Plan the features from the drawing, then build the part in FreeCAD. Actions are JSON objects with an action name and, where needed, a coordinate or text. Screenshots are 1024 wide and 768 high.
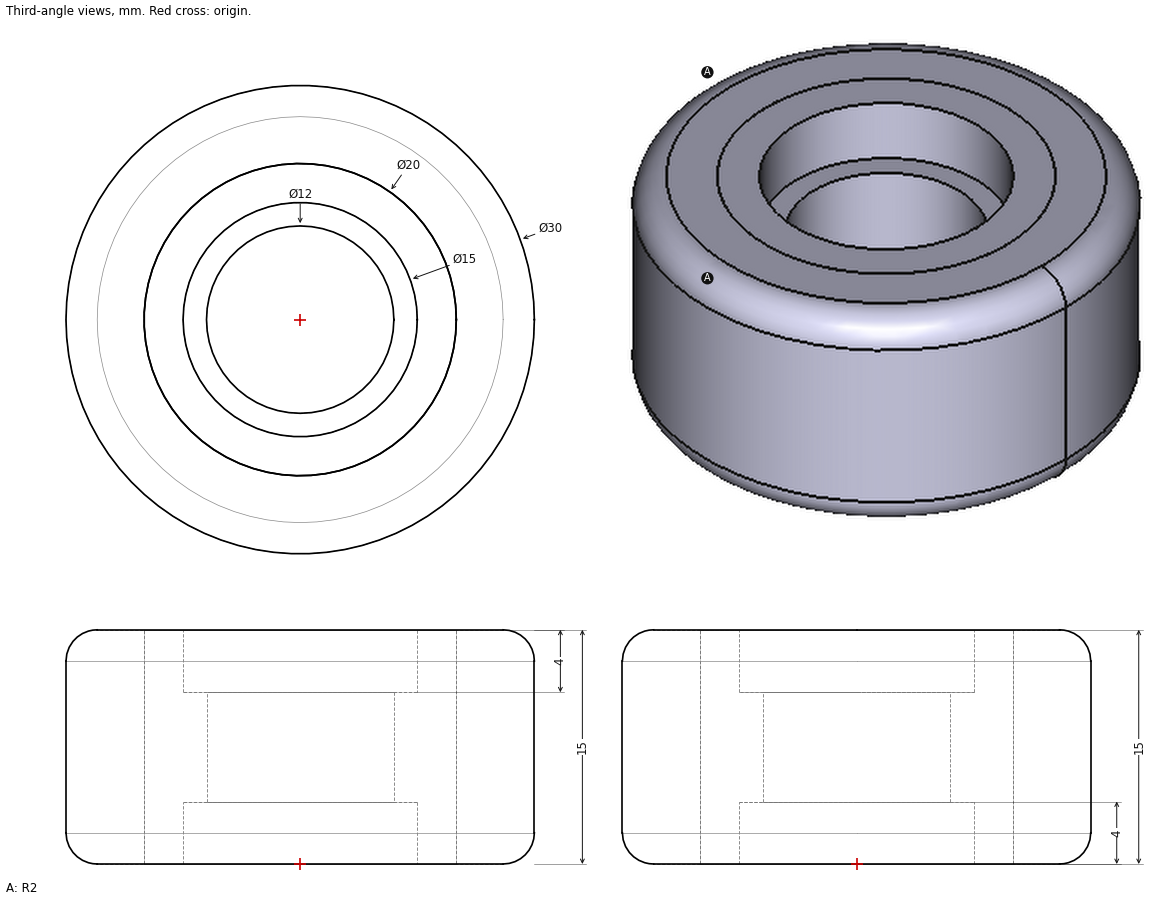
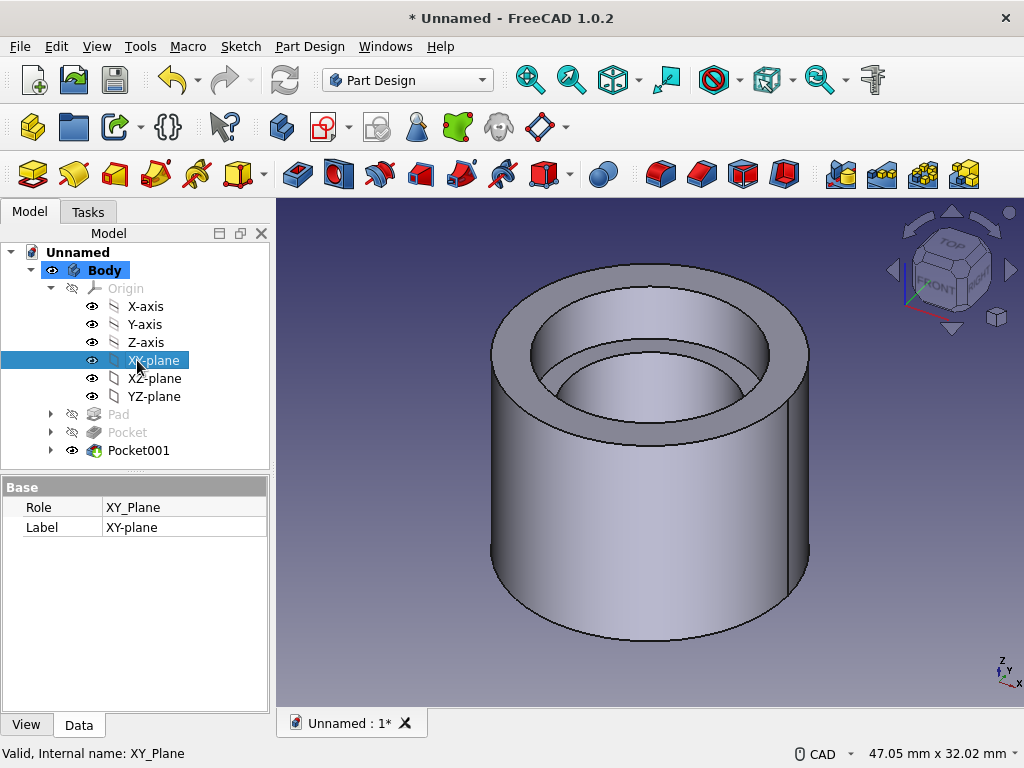
{"action": "left_click", "coordinate": [540, 128]}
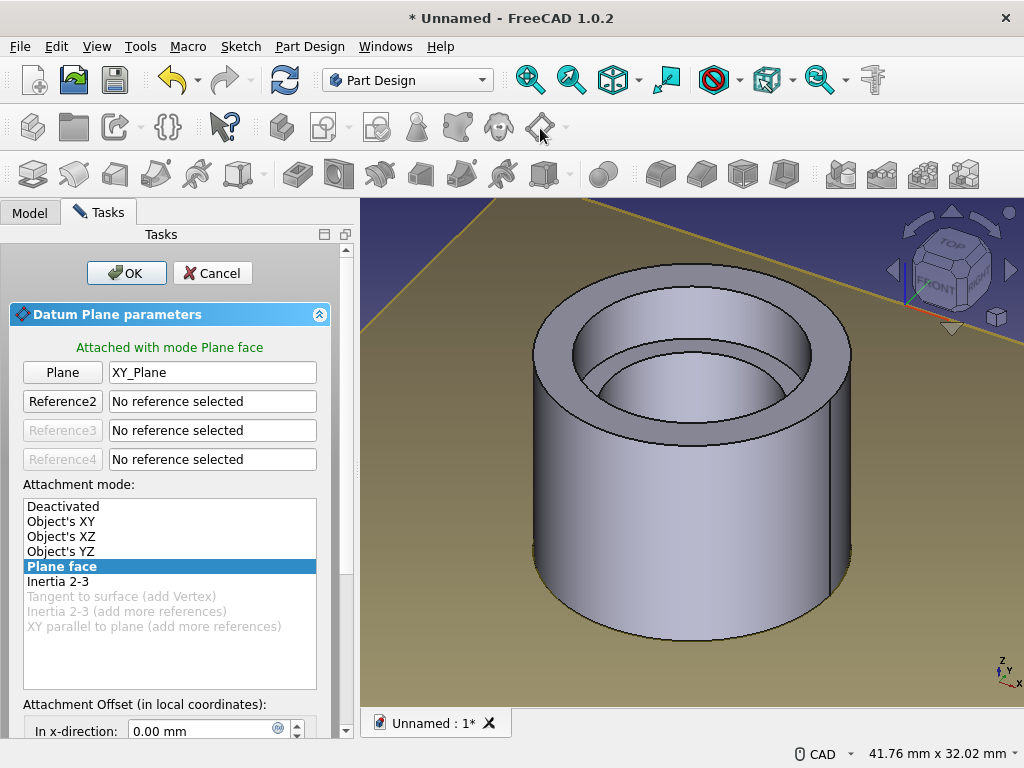
{"action": "scroll", "coordinate": [346, 491], "scroll_direction": "down", "scroll_amount": 3}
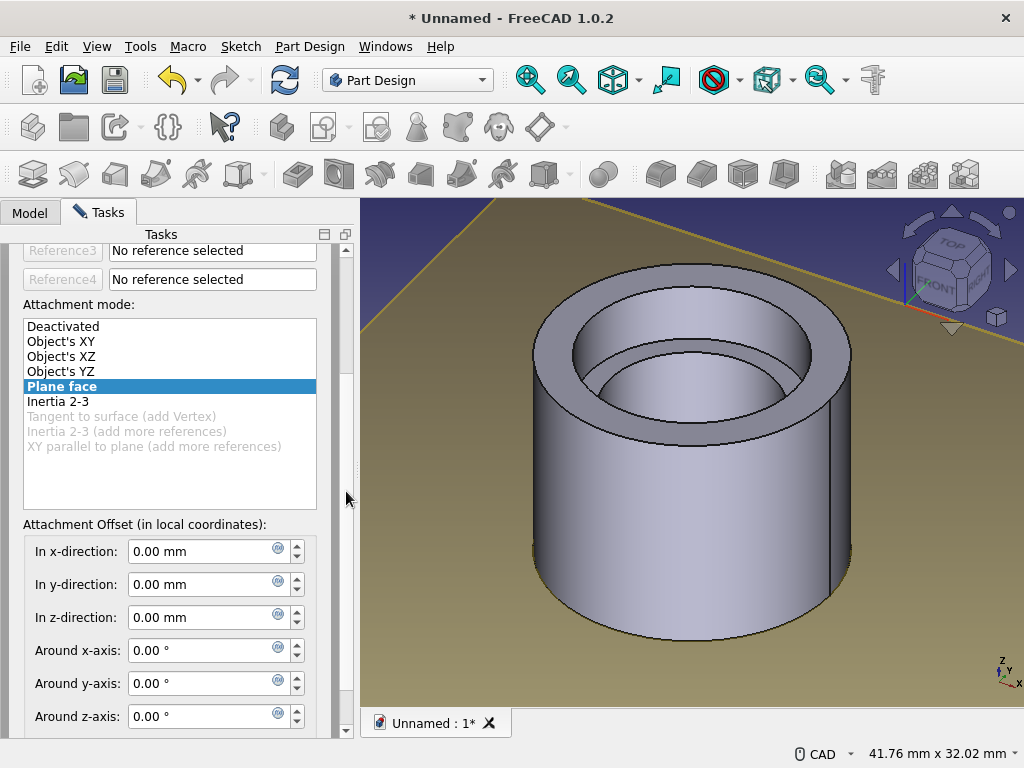
{"action": "triple_click", "coordinate": [210, 618]}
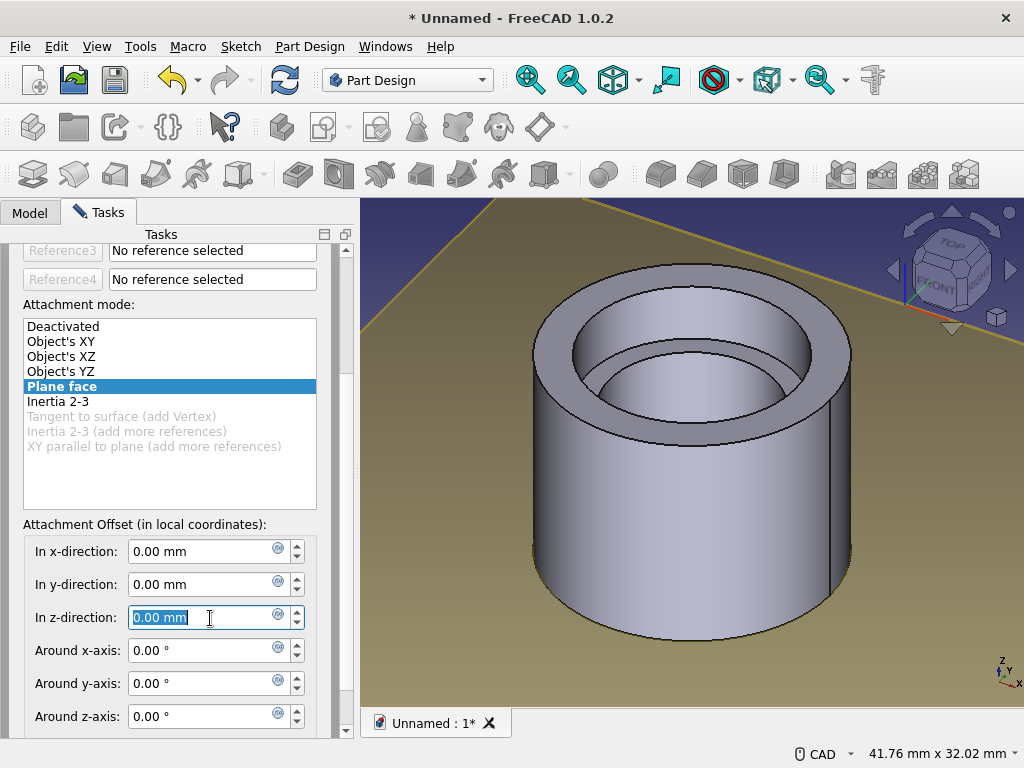
{"action": "type", "text": "4"}
{"action": "key", "text": "Tab"}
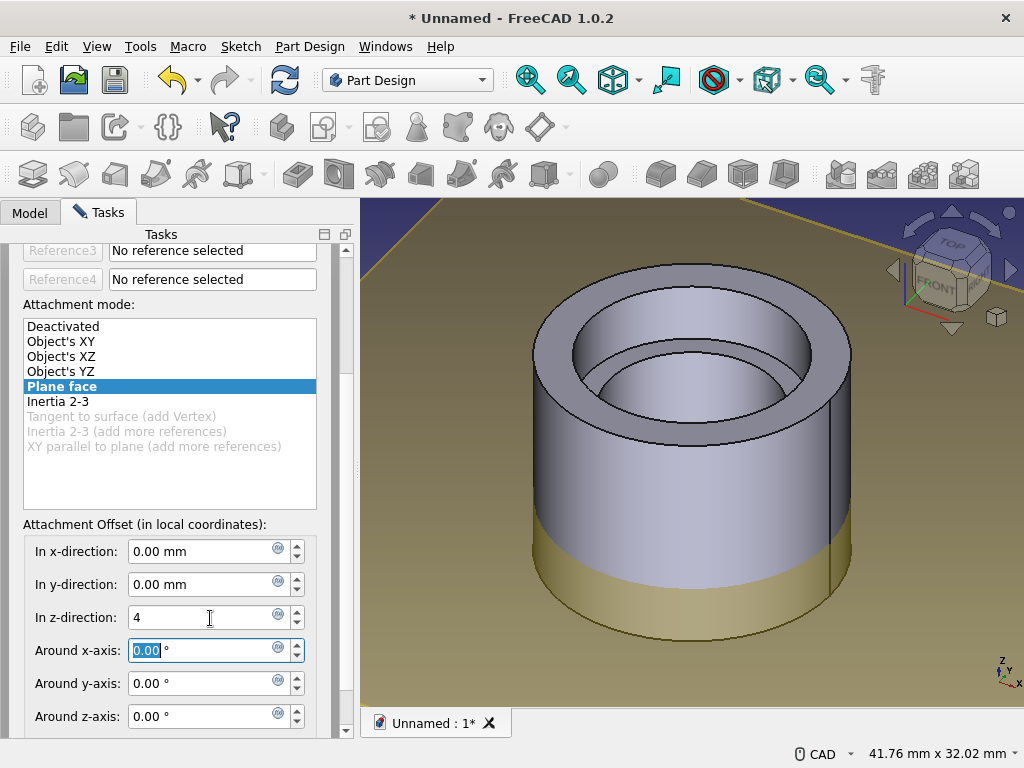
{"action": "scroll", "coordinate": [346, 491], "scroll_direction": "up", "scroll_amount": 4}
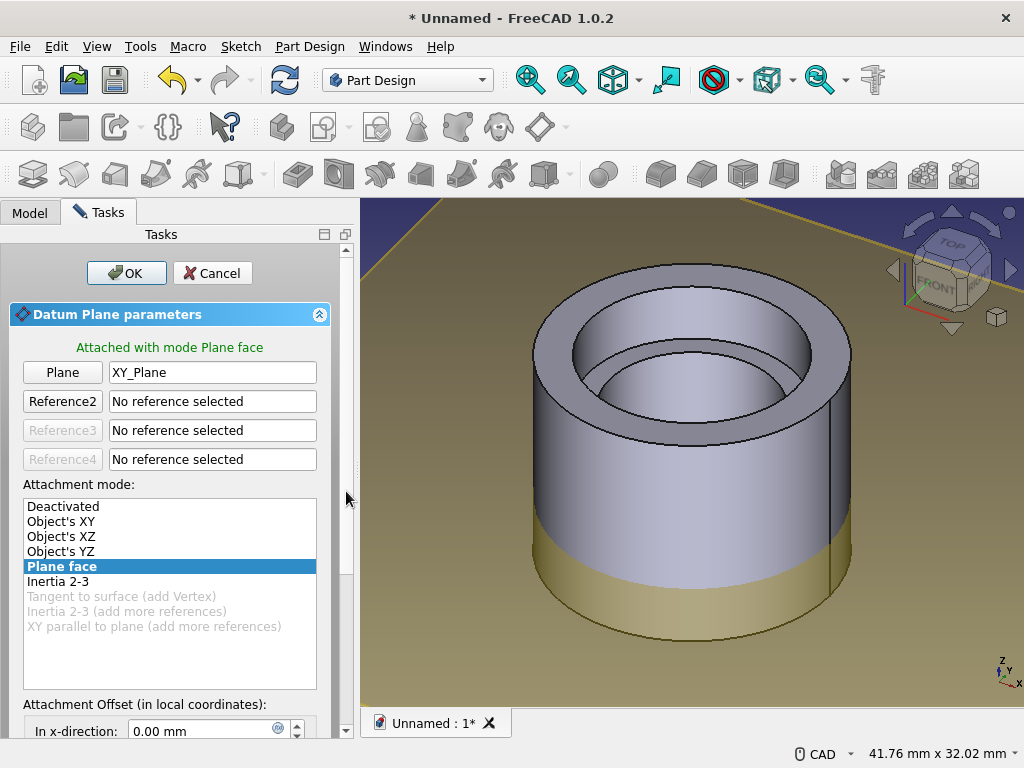
{"action": "left_click", "coordinate": [127, 273]}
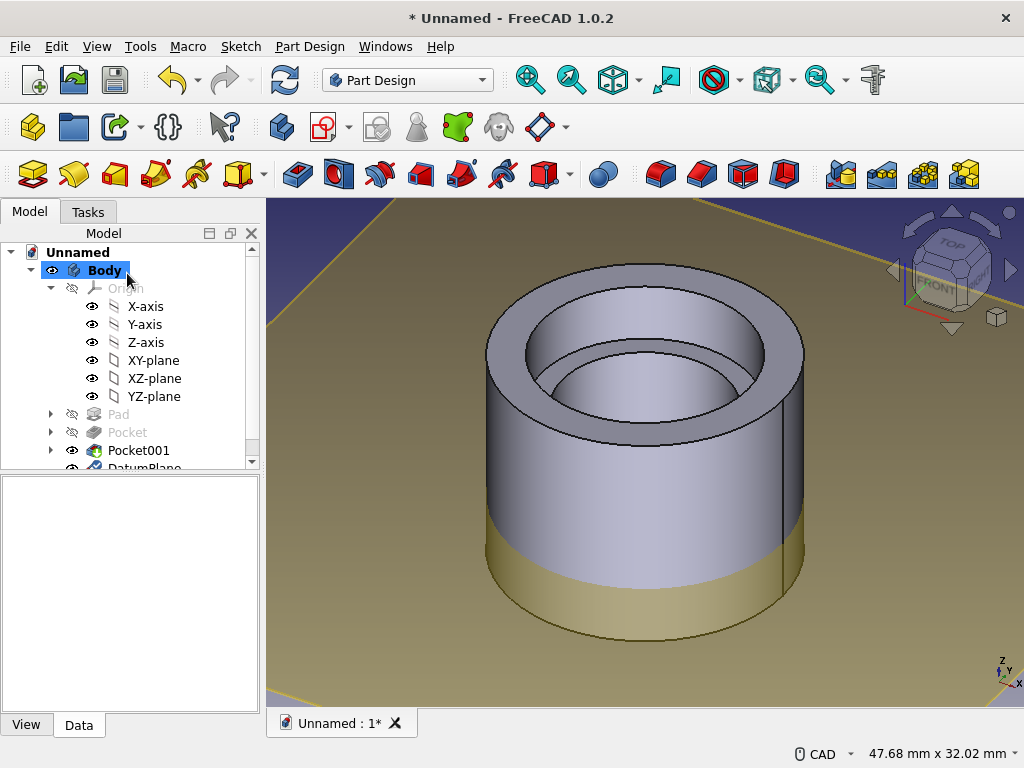
{"action": "left_click", "coordinate": [117, 468]}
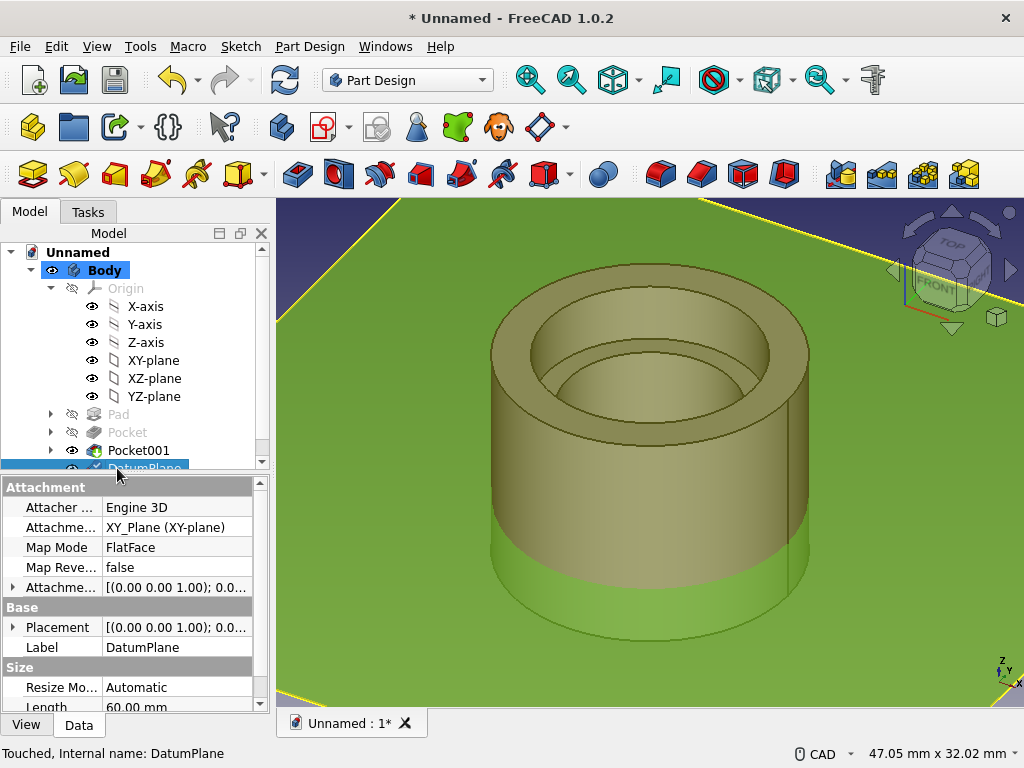
{"action": "left_click", "coordinate": [322, 128]}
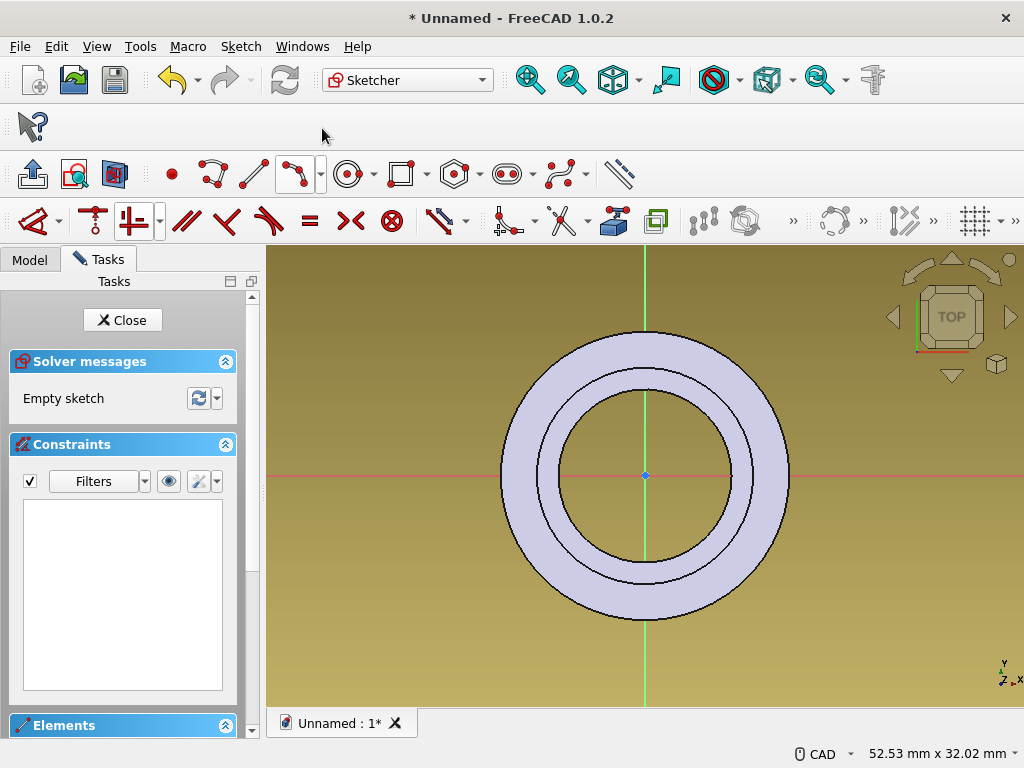
{"action": "key", "text": "q s"}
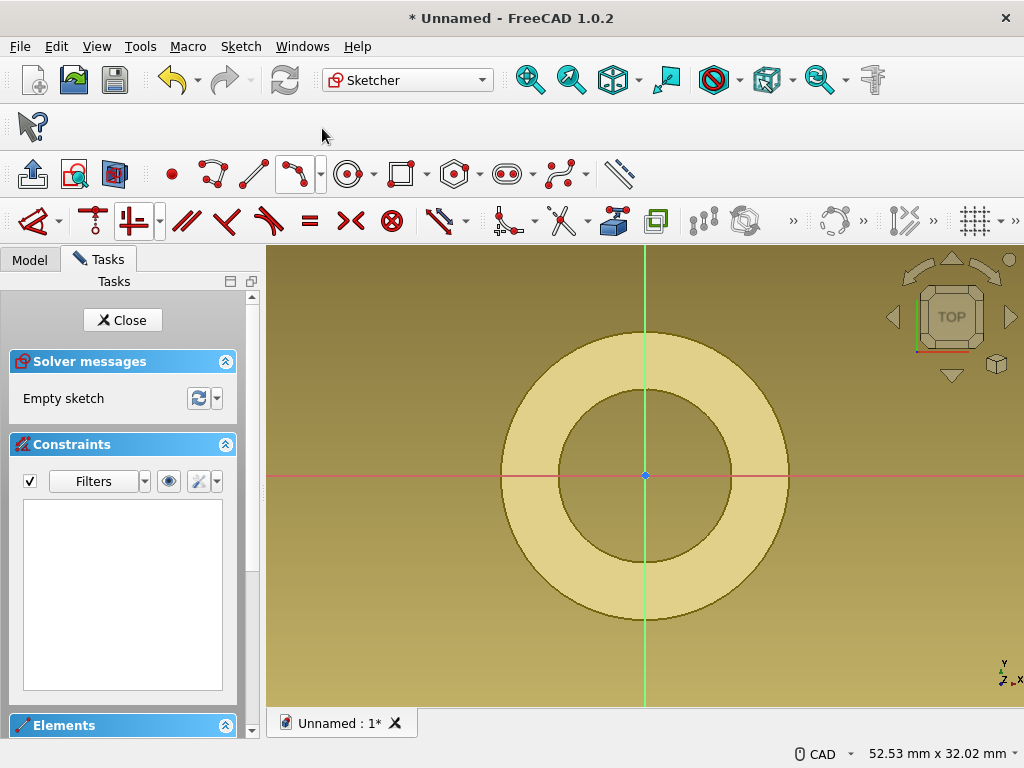
{"action": "left_click", "coordinate": [348, 174]}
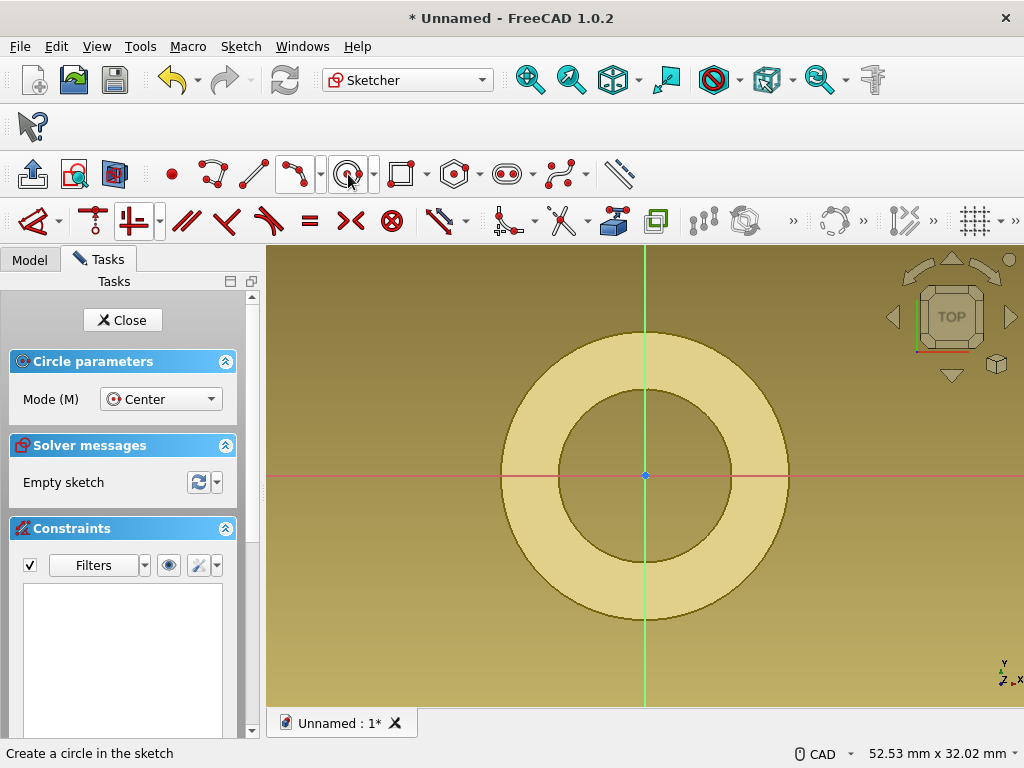
{"action": "left_click", "coordinate": [645, 476]}
{"action": "mouse_move", "coordinate": [722, 399]}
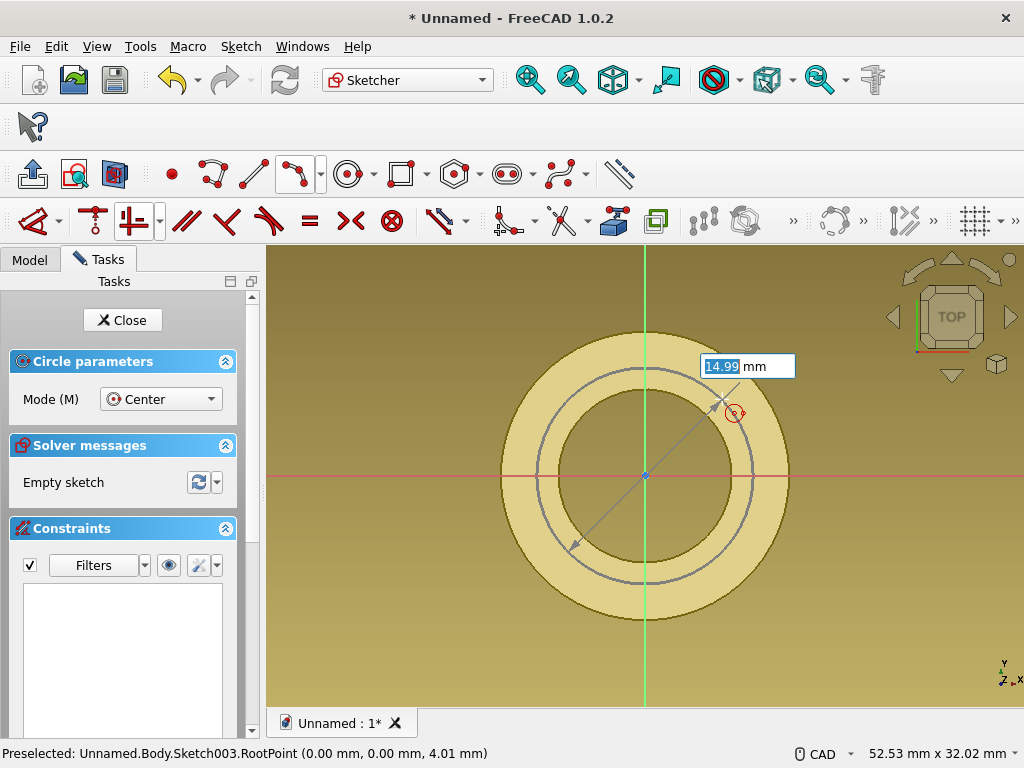
{"action": "type", "text": "15"}
{"action": "key", "text": "Return"}
{"action": "key", "text": "Escape"}